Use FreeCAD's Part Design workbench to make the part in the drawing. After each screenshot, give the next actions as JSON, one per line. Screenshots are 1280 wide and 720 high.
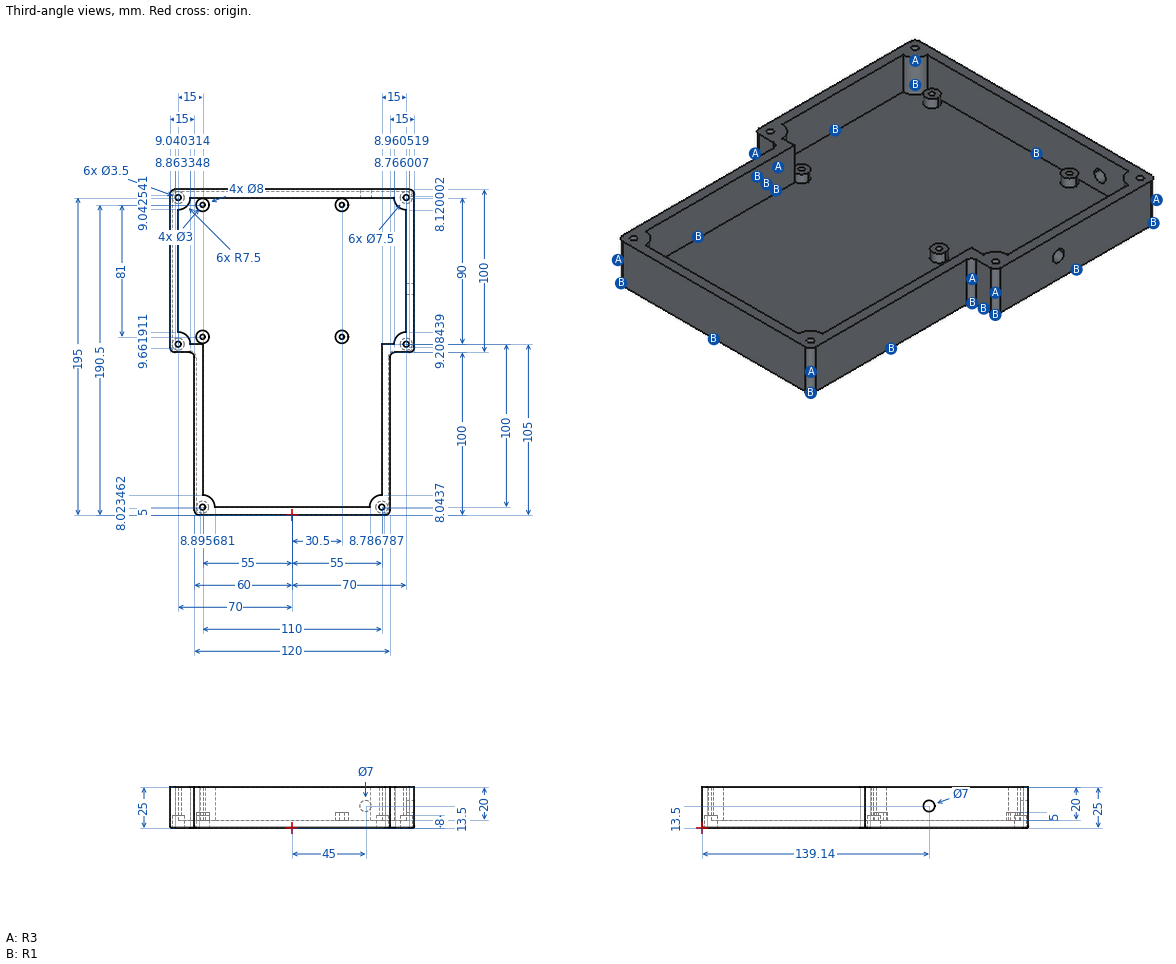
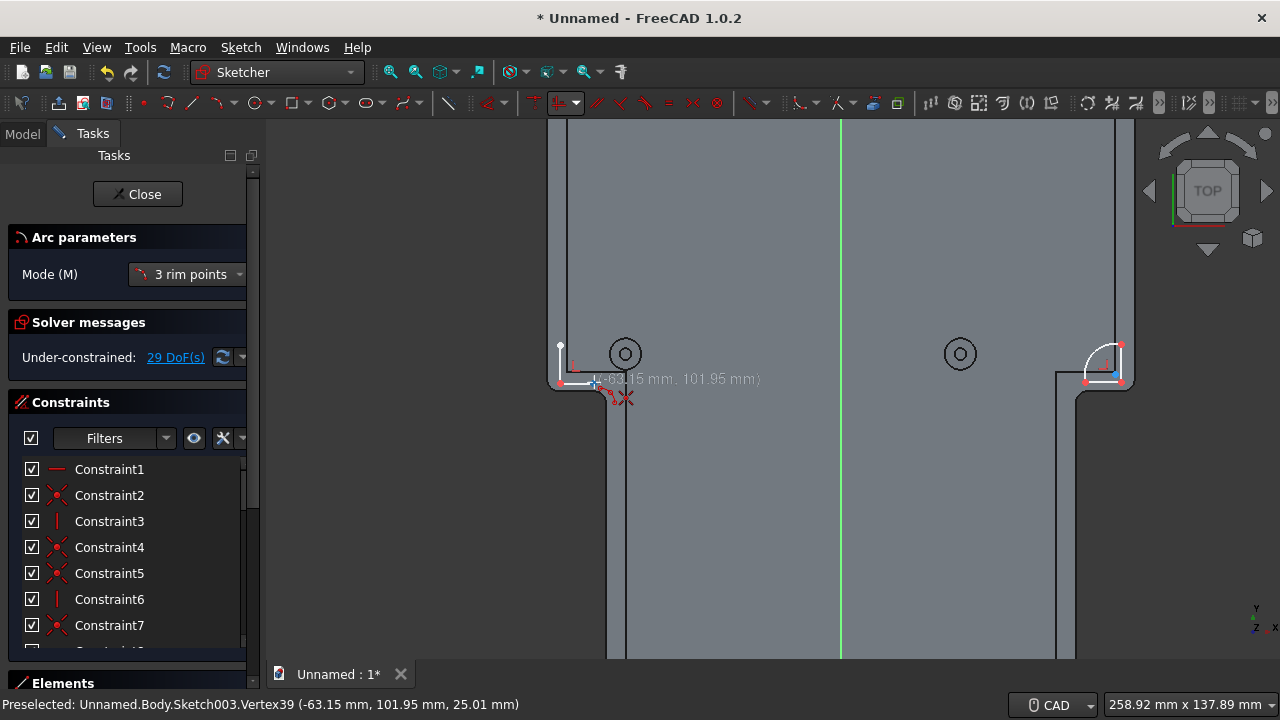
{"action": "left_click", "coordinate": [594, 384]}
{"action": "left_click", "coordinate": [560, 346]}
{"action": "left_click", "coordinate": [588, 352]}
{"action": "key", "text": "Escape"}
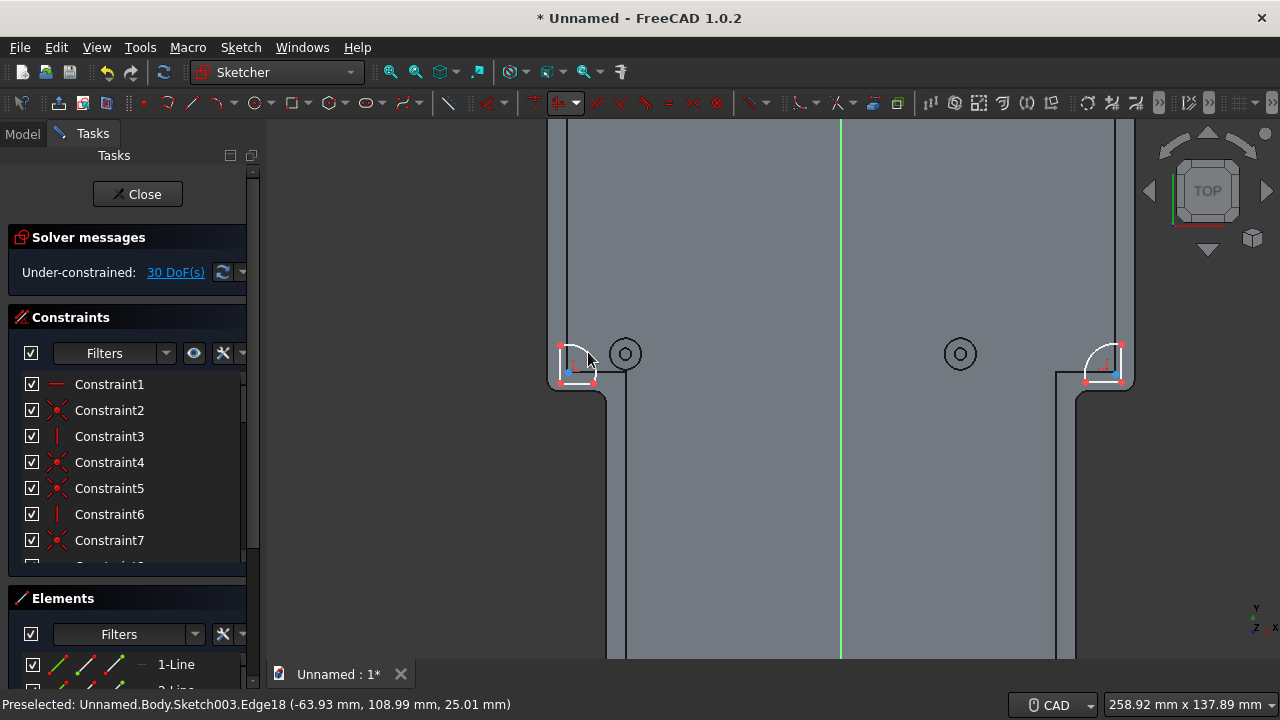
{"action": "scroll", "coordinate": [594, 382], "scroll_direction": "down", "scroll_amount": 4}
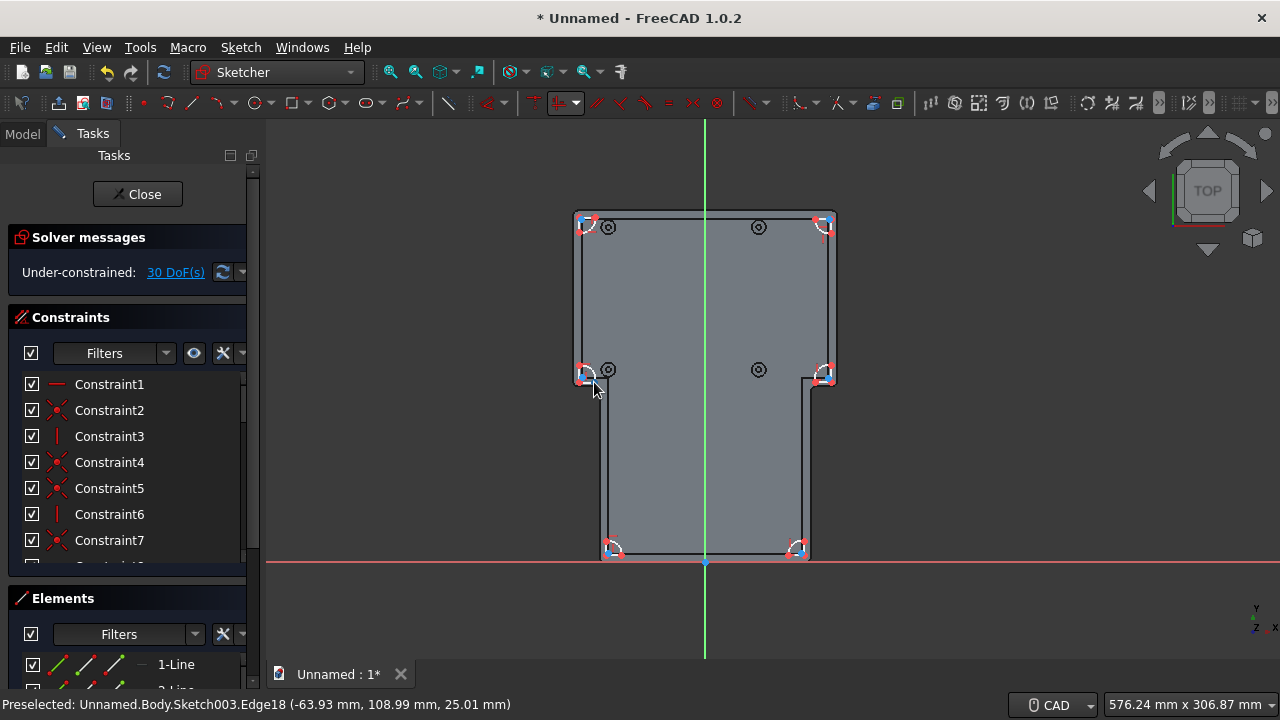
{"action": "scroll", "coordinate": [587, 232], "scroll_direction": "up", "scroll_amount": 4}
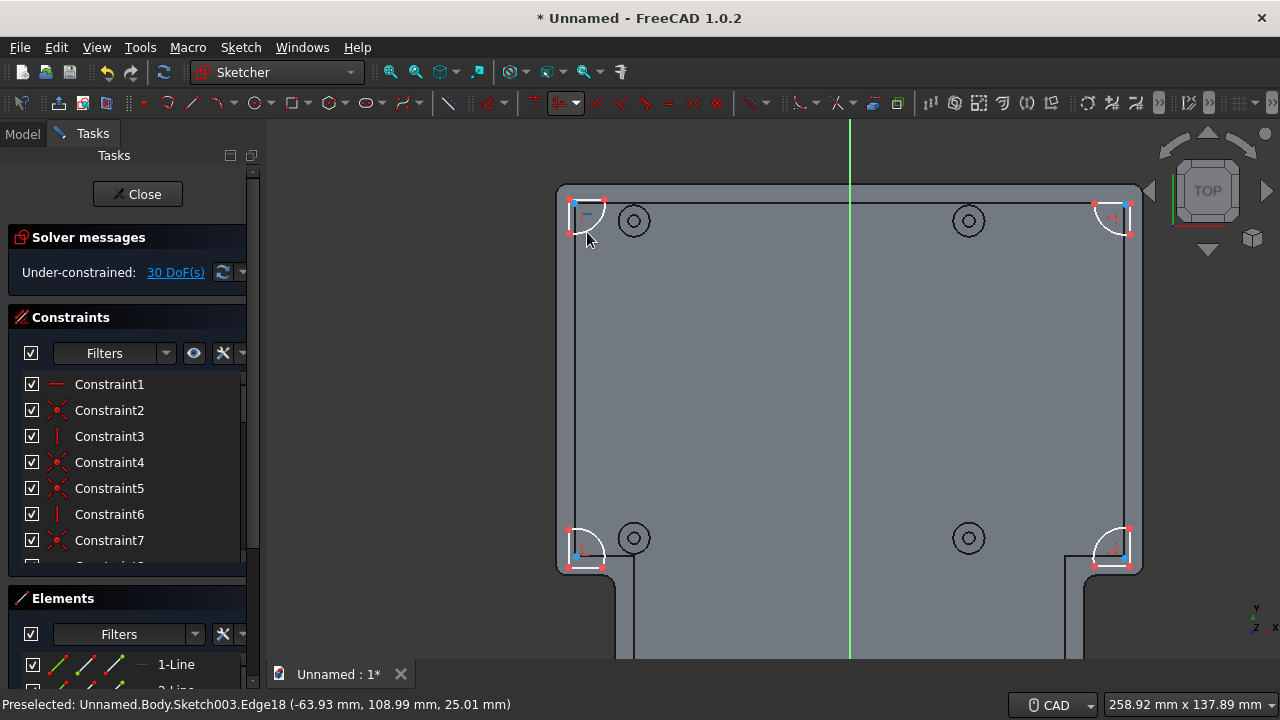
{"action": "left_click", "coordinate": [586, 231]}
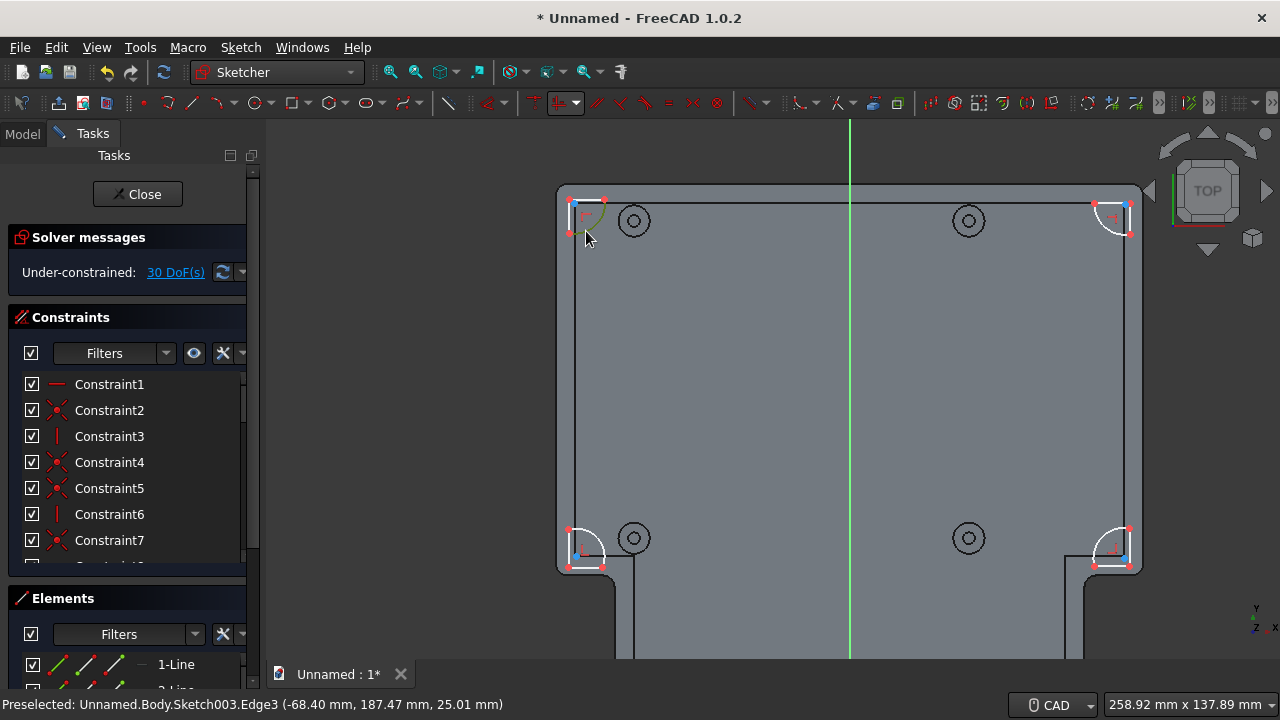
{"action": "left_click", "coordinate": [1098, 219]}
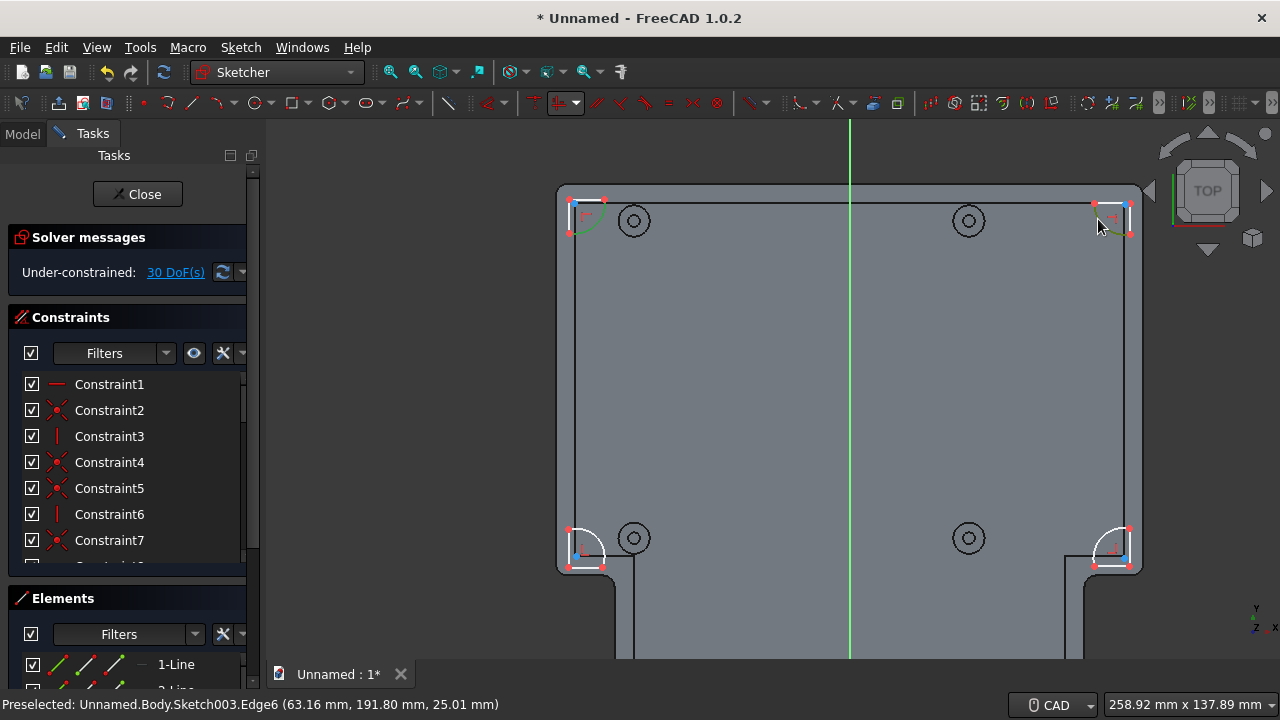
{"action": "left_click", "coordinate": [1112, 530]}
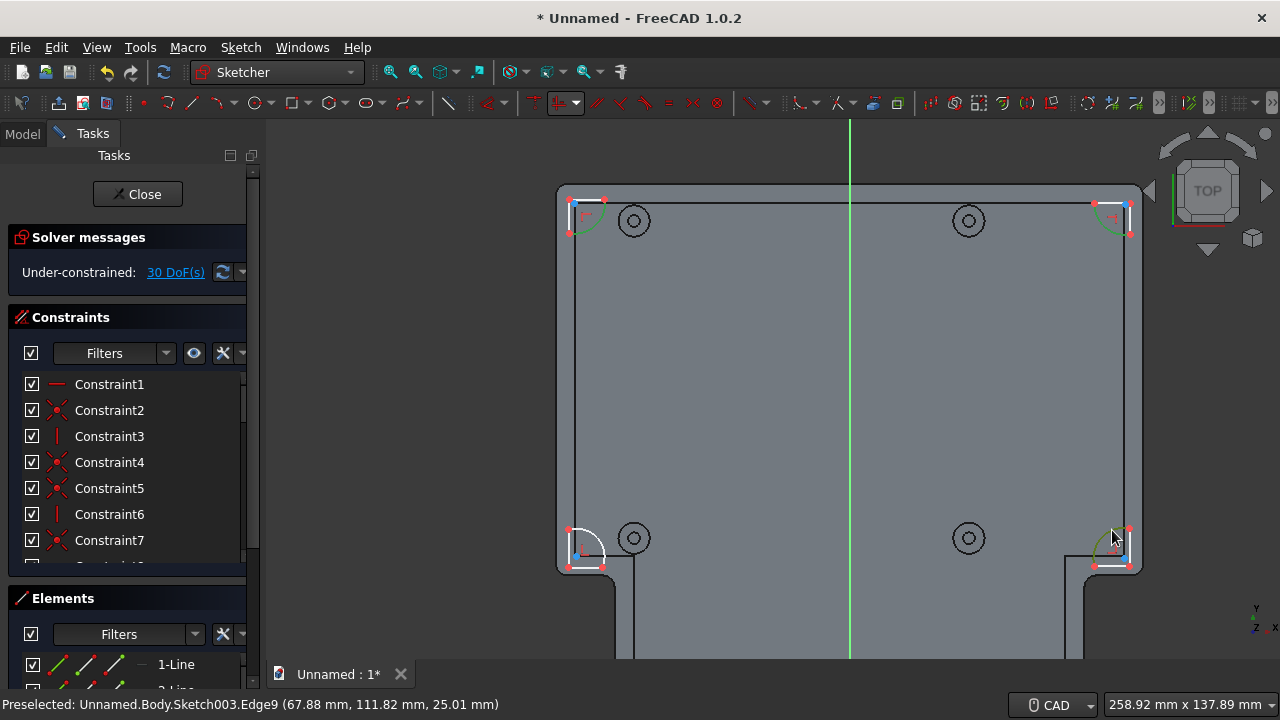
{"action": "scroll", "coordinate": [587, 232], "scroll_direction": "down", "scroll_amount": 4}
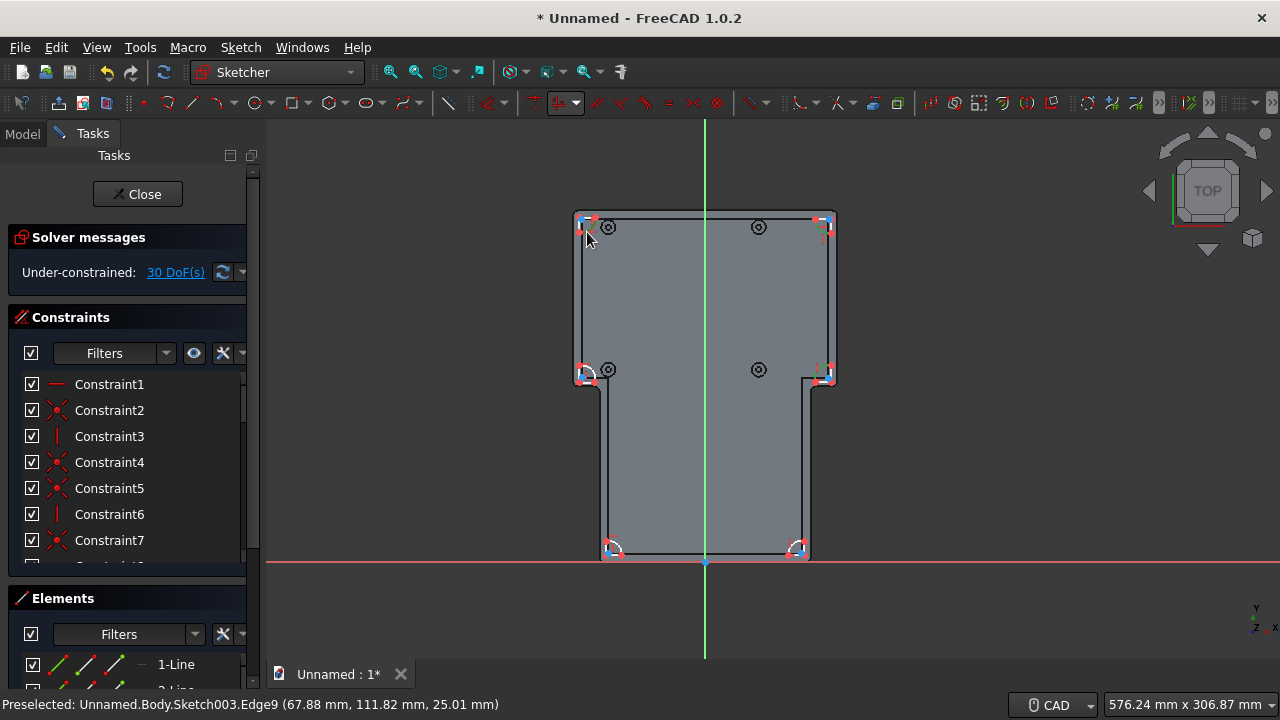
{"action": "scroll", "coordinate": [620, 548], "scroll_direction": "up", "scroll_amount": 4}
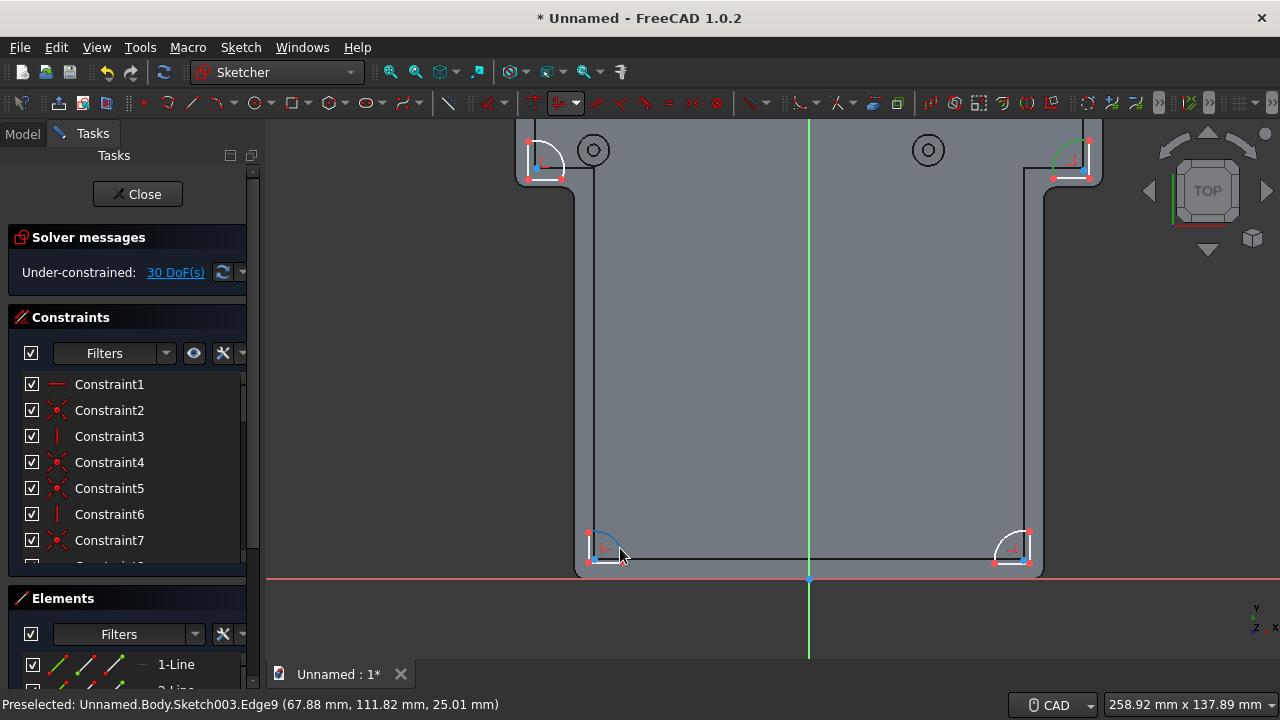
{"action": "left_click", "coordinate": [620, 547]}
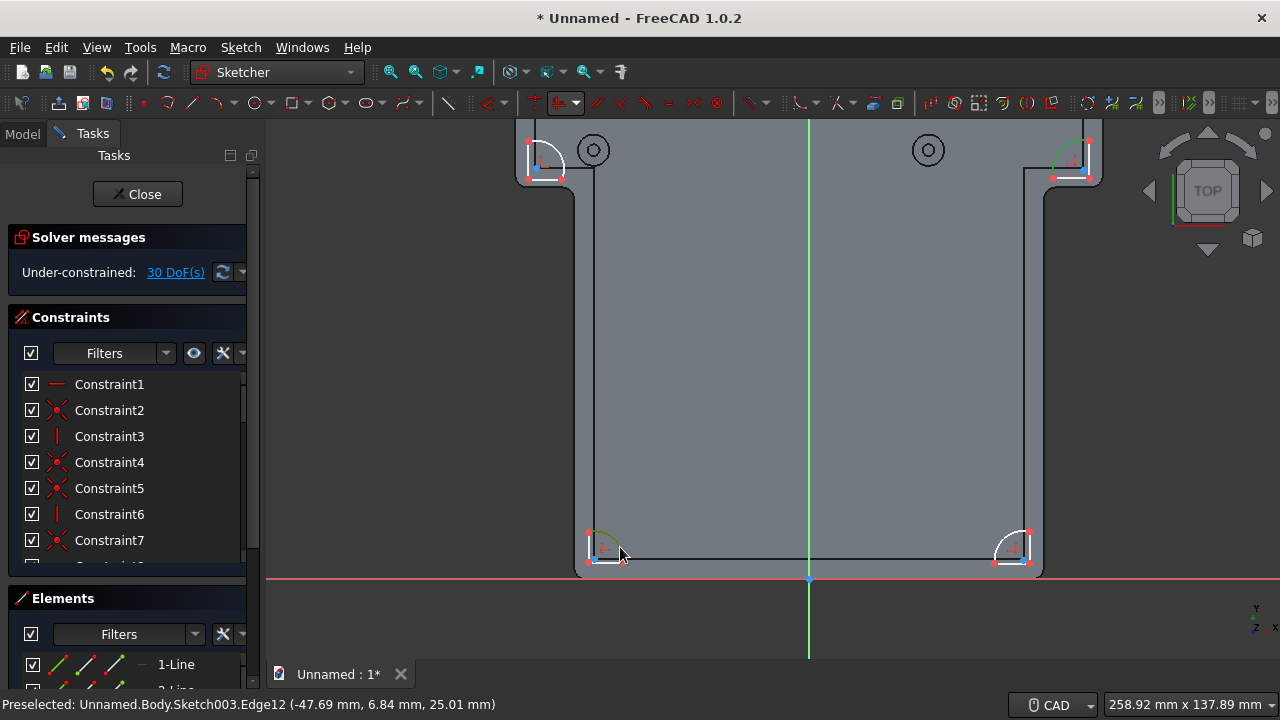
{"action": "left_click", "coordinate": [1013, 533]}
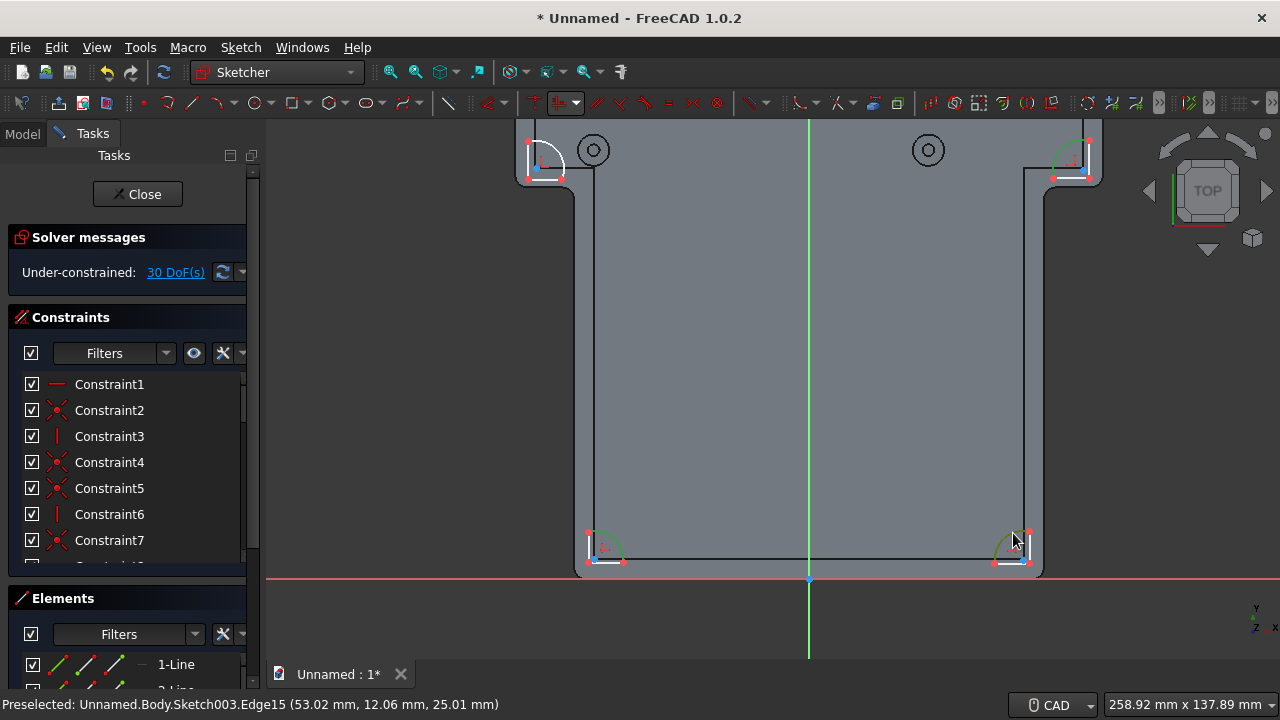
{"action": "left_click", "coordinate": [563, 161]}